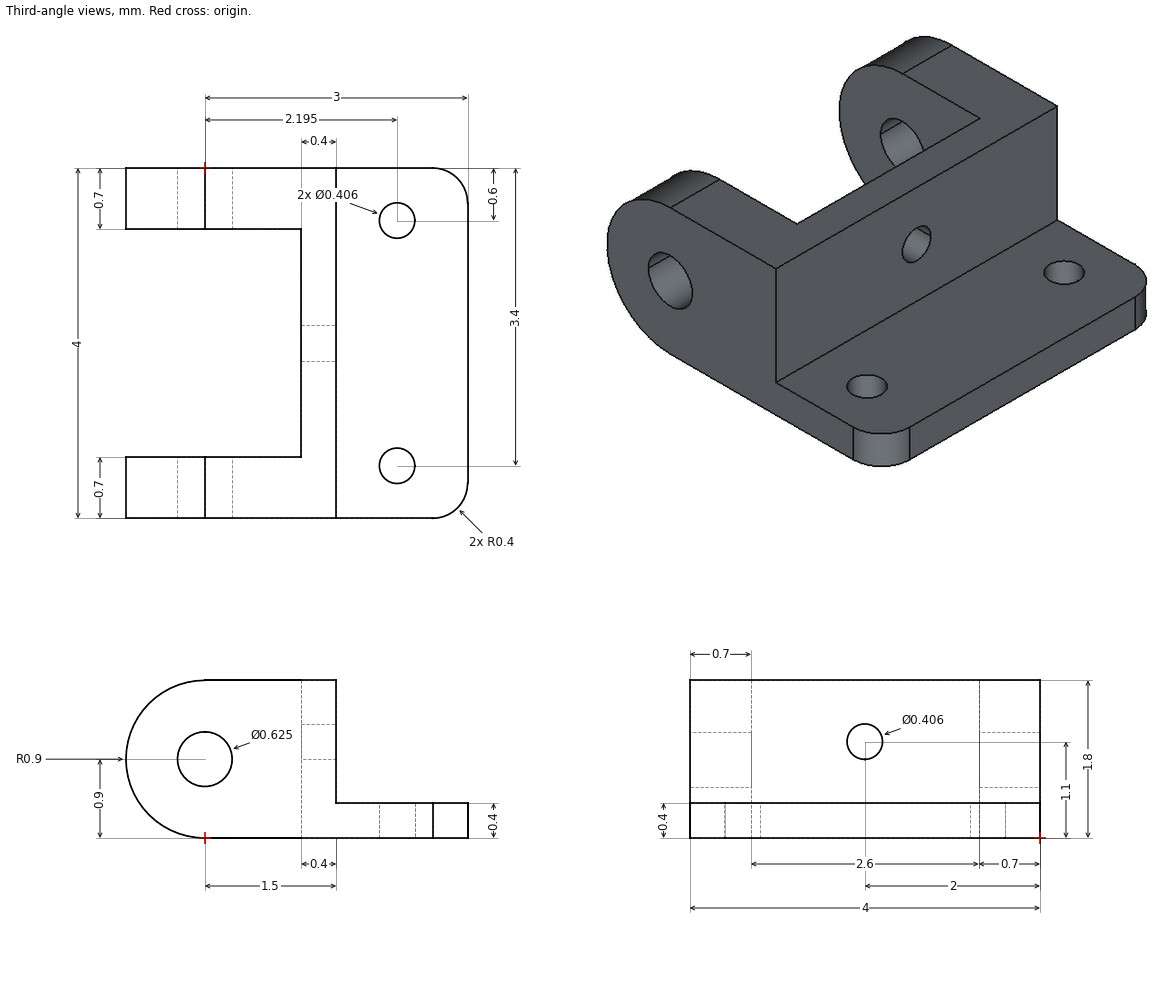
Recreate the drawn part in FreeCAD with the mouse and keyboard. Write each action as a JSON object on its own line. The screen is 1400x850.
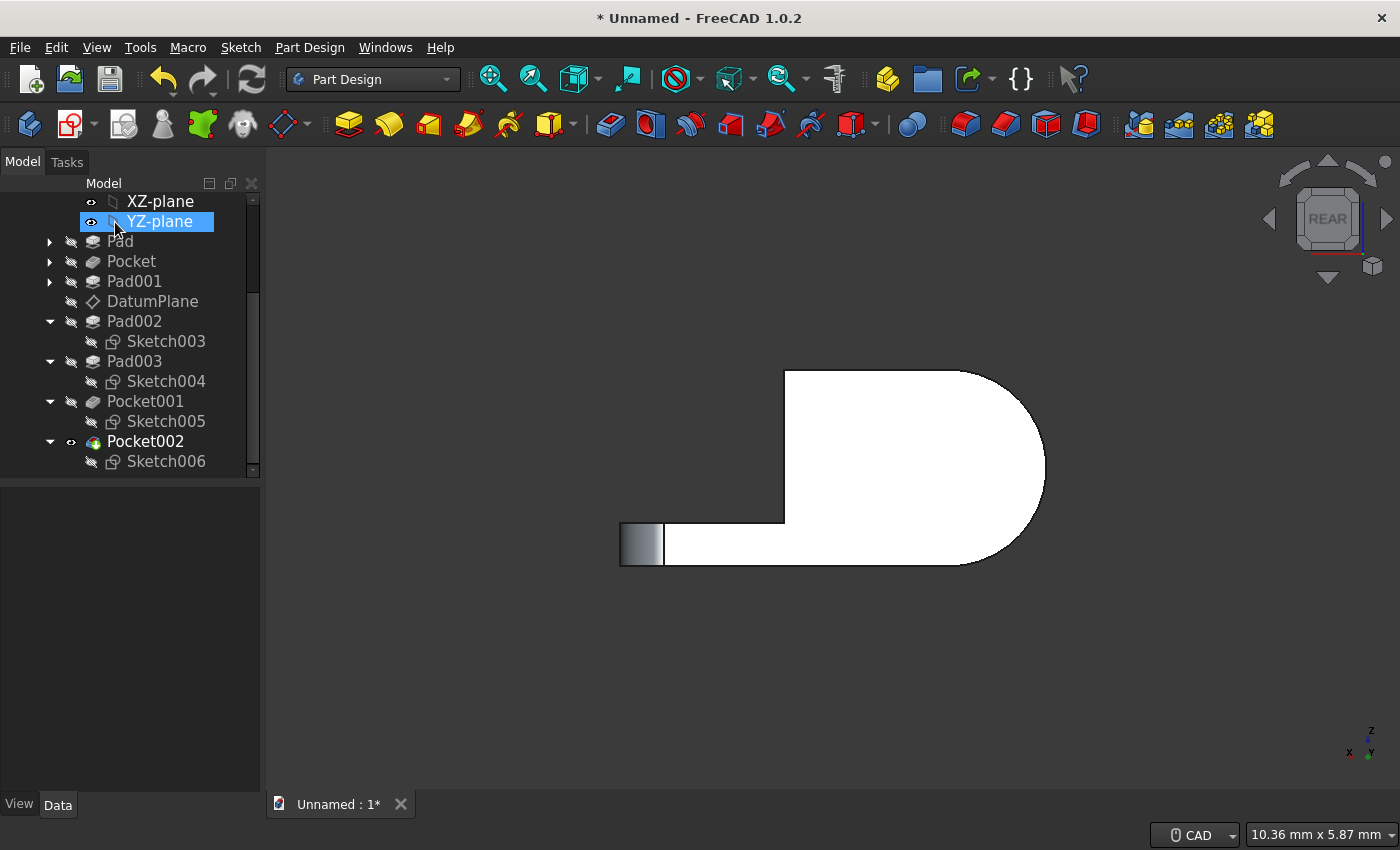
{"action": "left_click", "coordinate": [494, 80]}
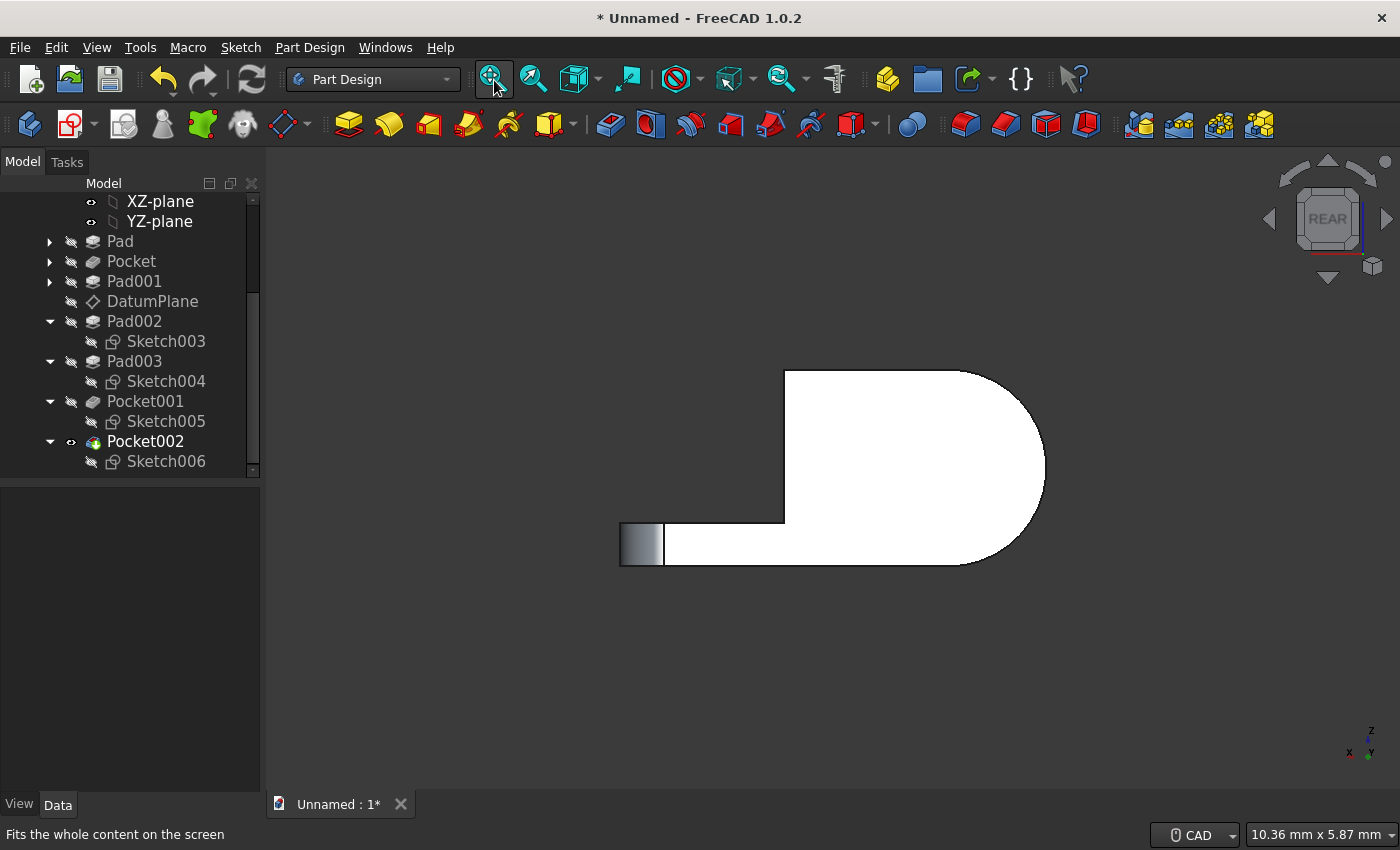
{"action": "left_click", "coordinate": [910, 467]}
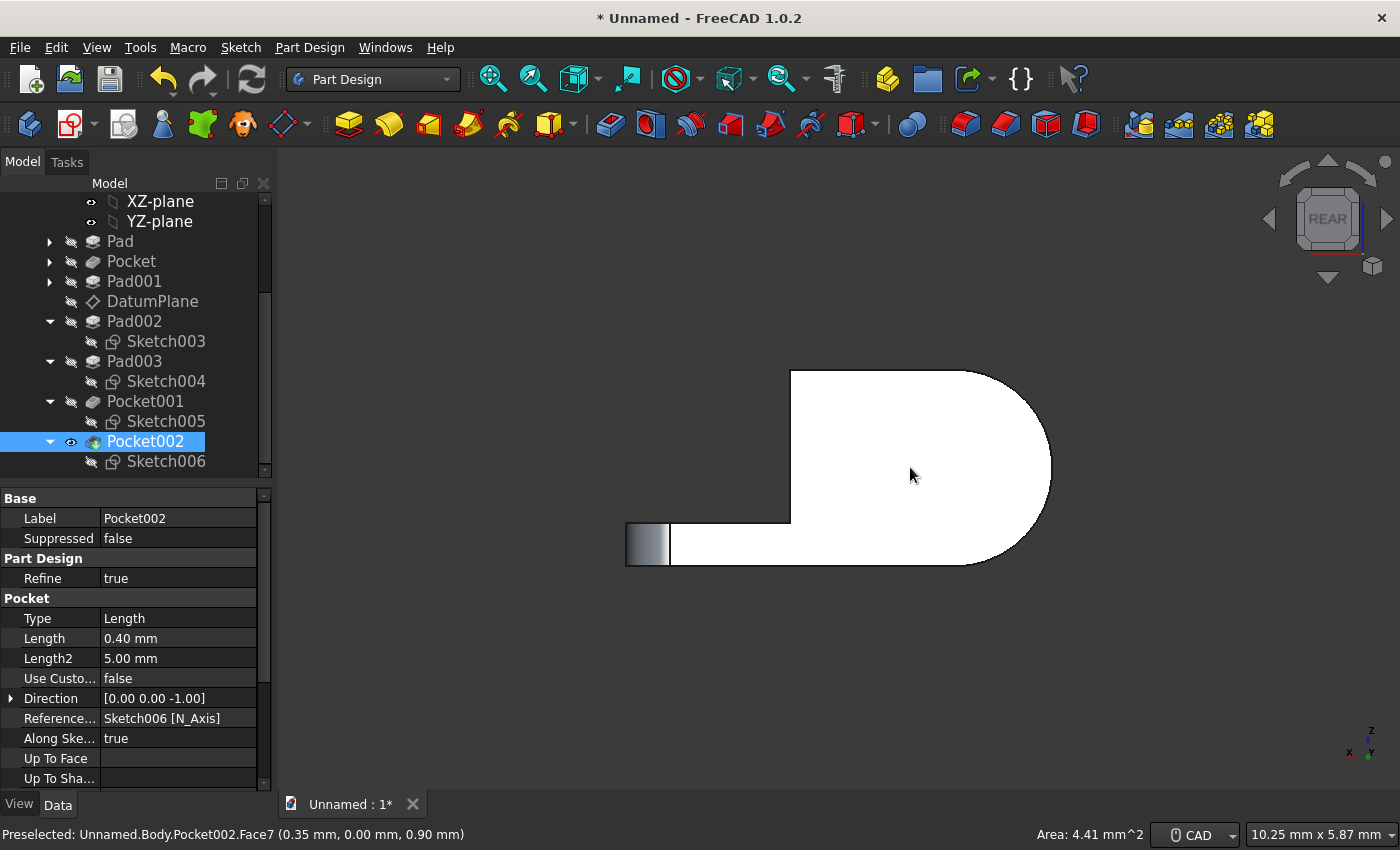
{"action": "left_click", "coordinate": [70, 124]}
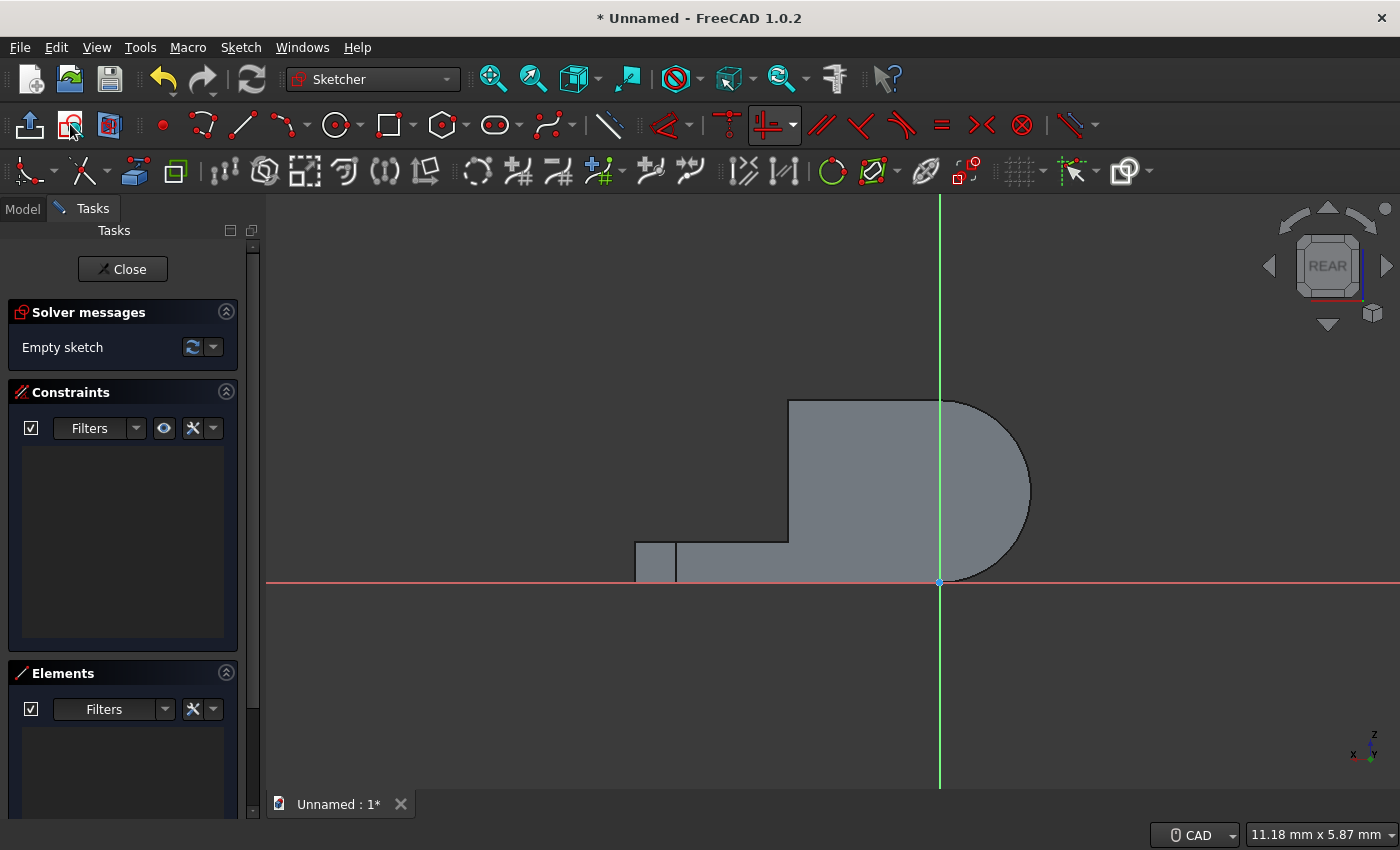
{"action": "scroll", "coordinate": [1015, 534], "scroll_direction": "up", "scroll_amount": 6}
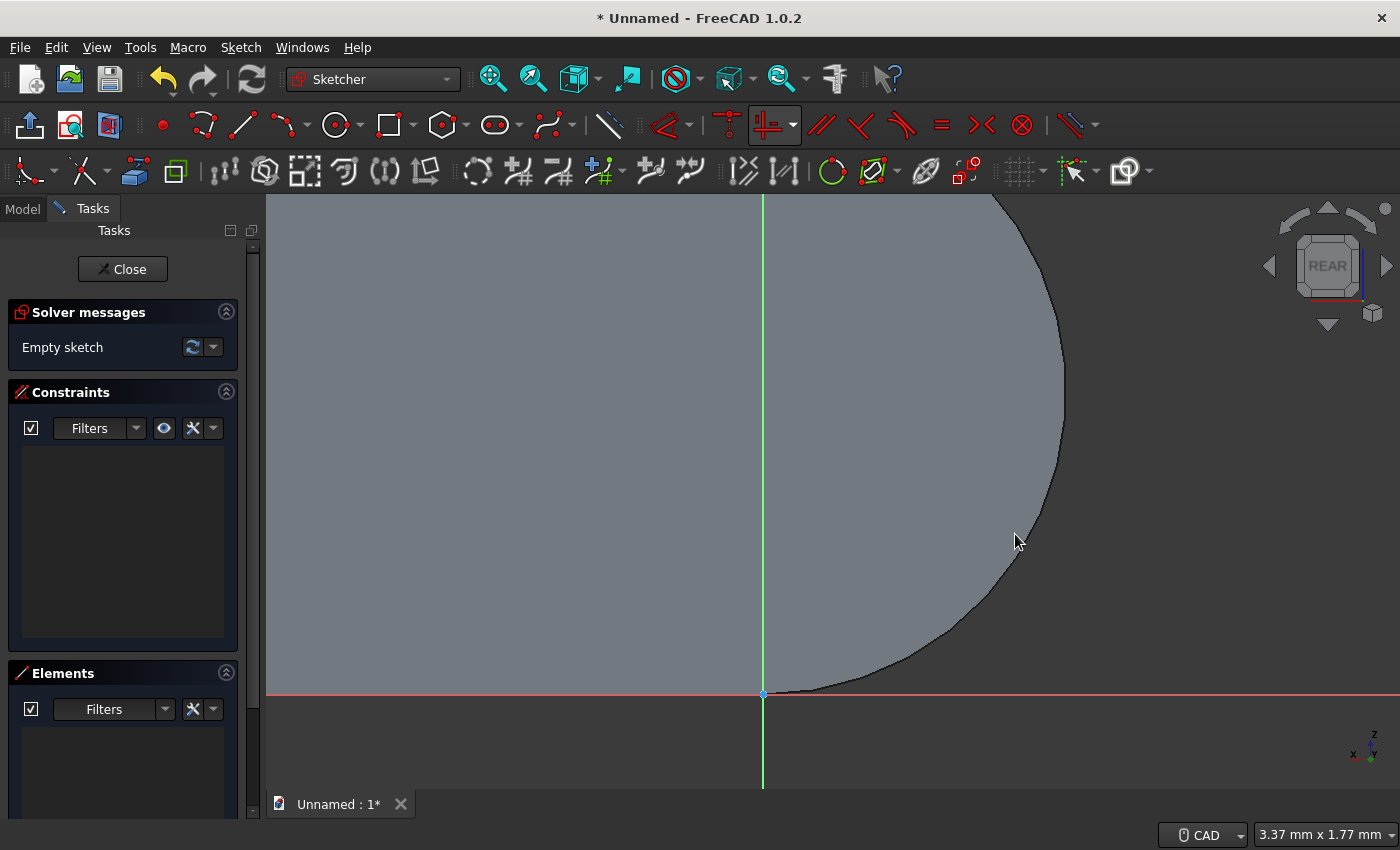
{"action": "key", "text": "g c"}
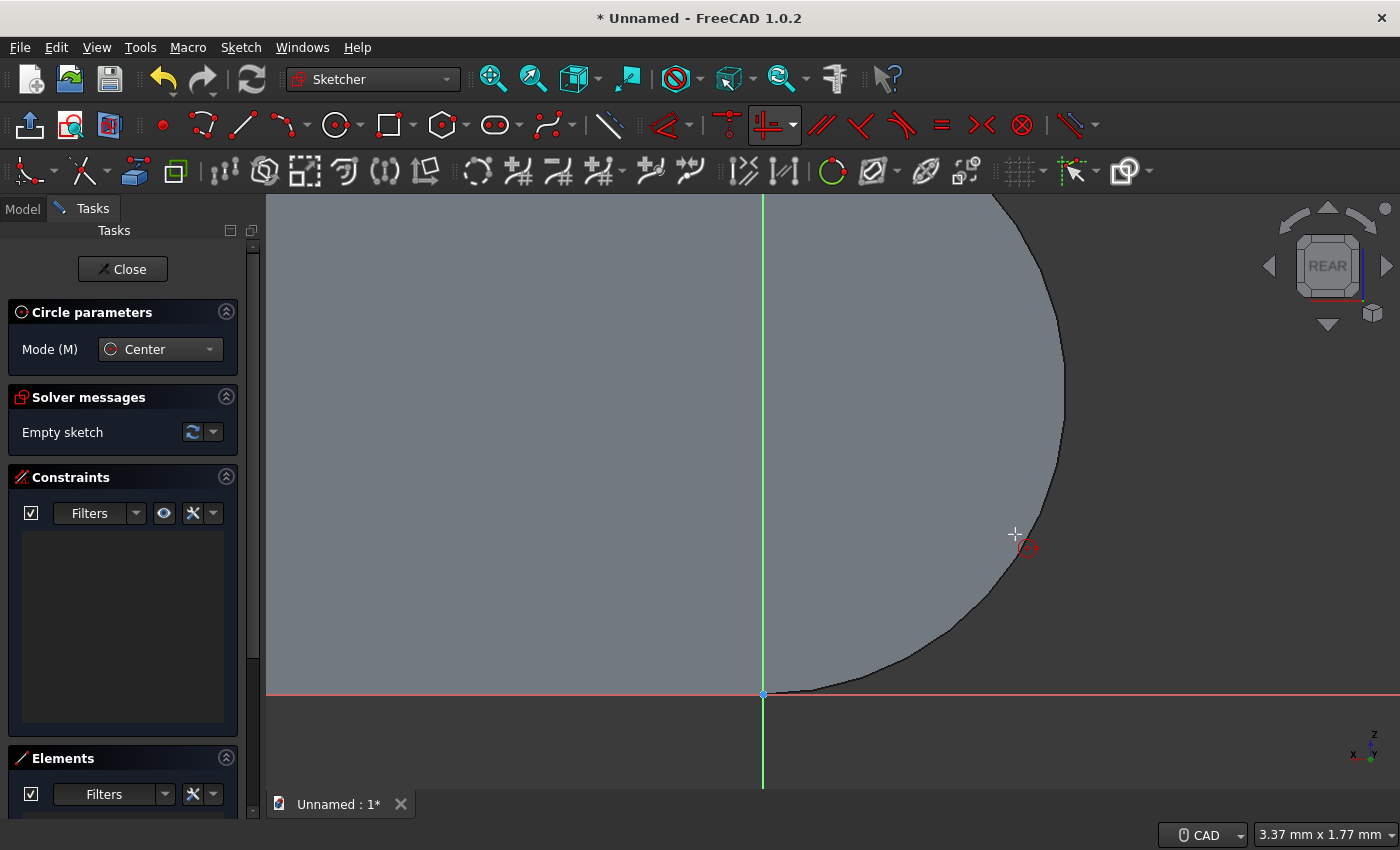
{"action": "left_click", "coordinate": [763, 392]}
{"action": "mouse_move", "coordinate": [838, 317]}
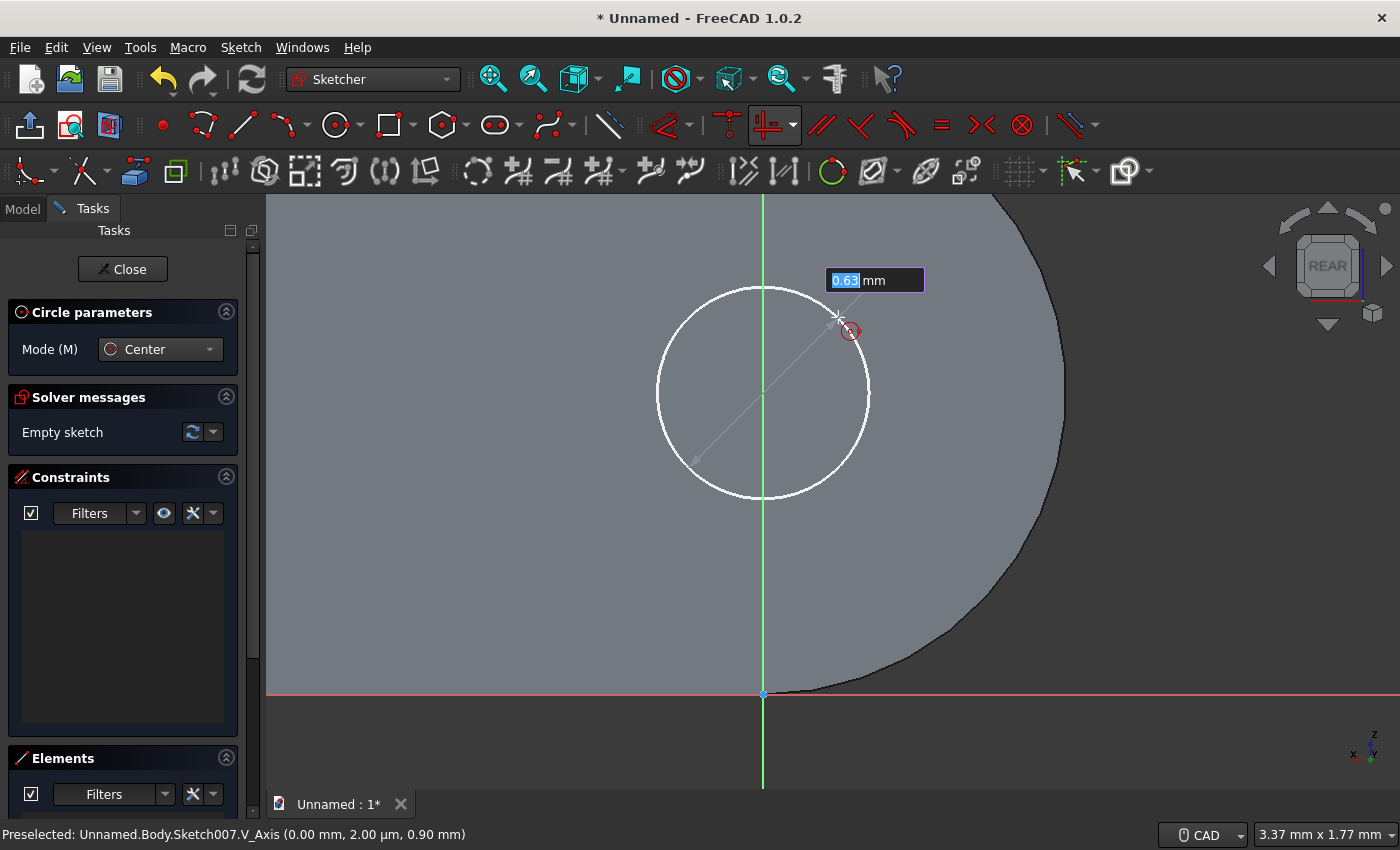
{"action": "type", "text": "0.625"}
{"action": "key", "text": "Return"}
{"action": "key", "text": "Escape"}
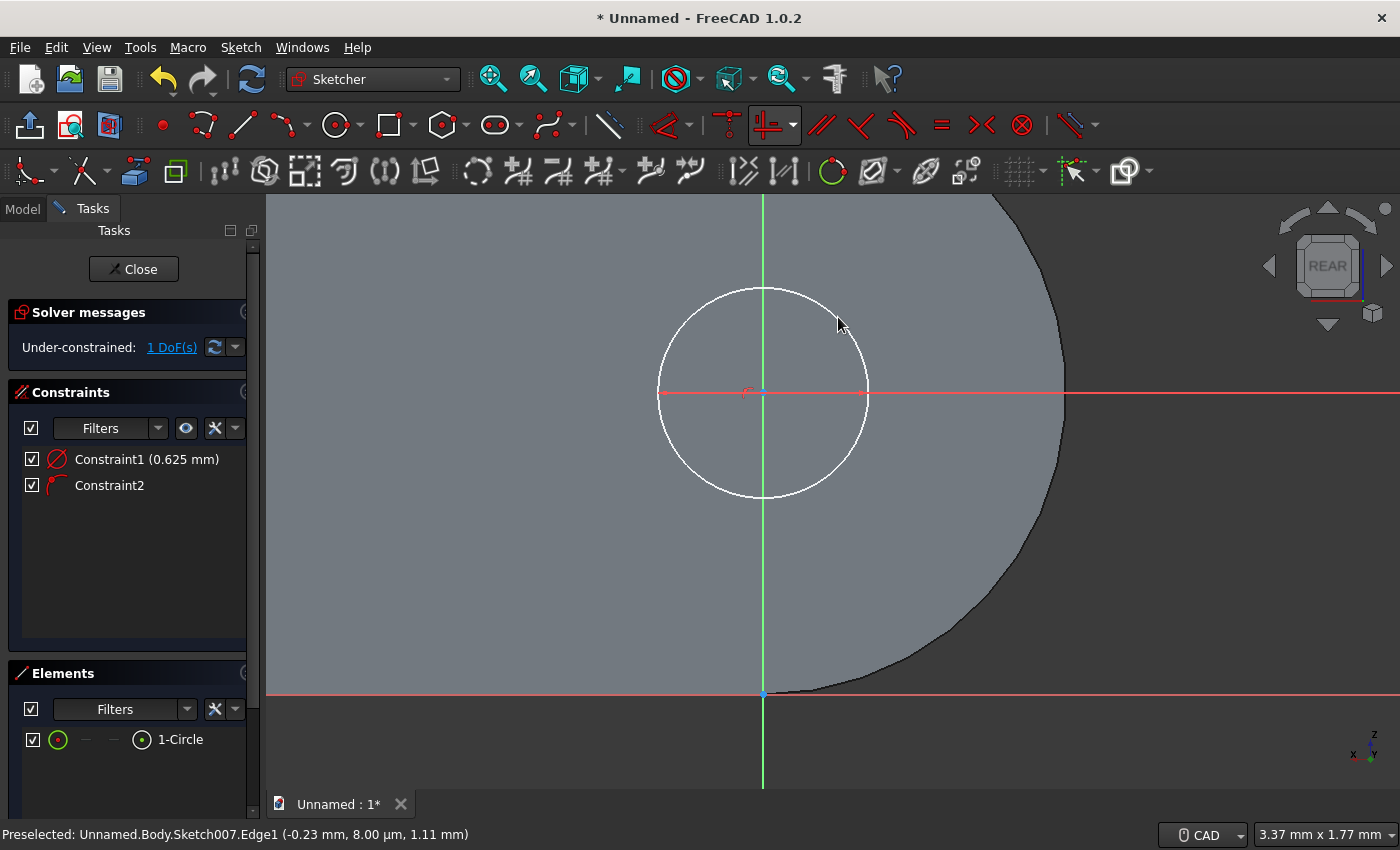
{"action": "left_click", "coordinate": [664, 126]}